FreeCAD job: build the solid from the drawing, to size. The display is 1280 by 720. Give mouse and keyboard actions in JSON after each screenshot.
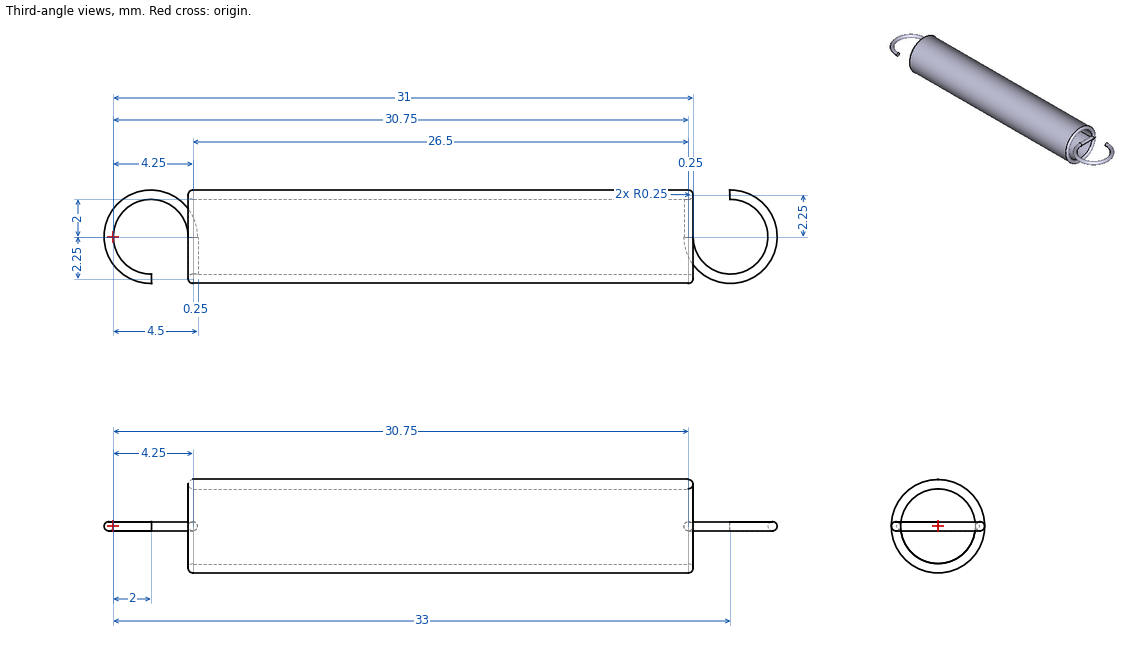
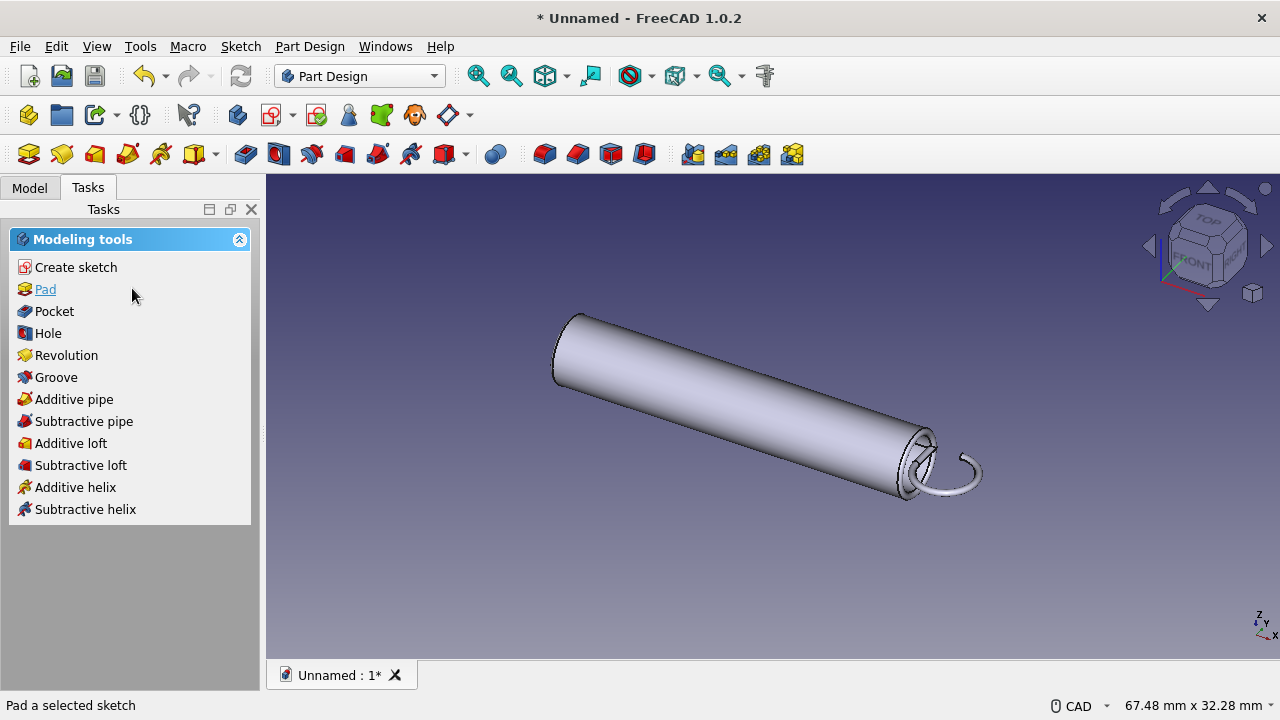
{"action": "left_click", "coordinate": [62, 154]}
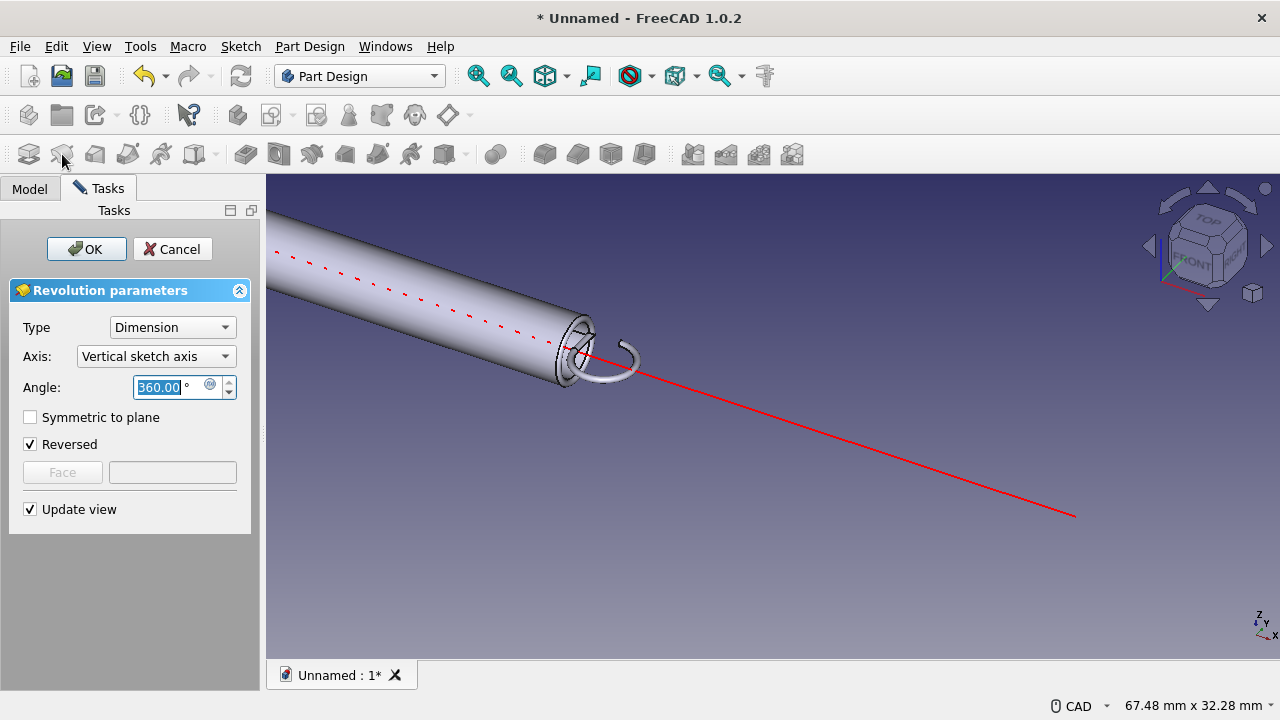
{"action": "left_click", "coordinate": [157, 356]}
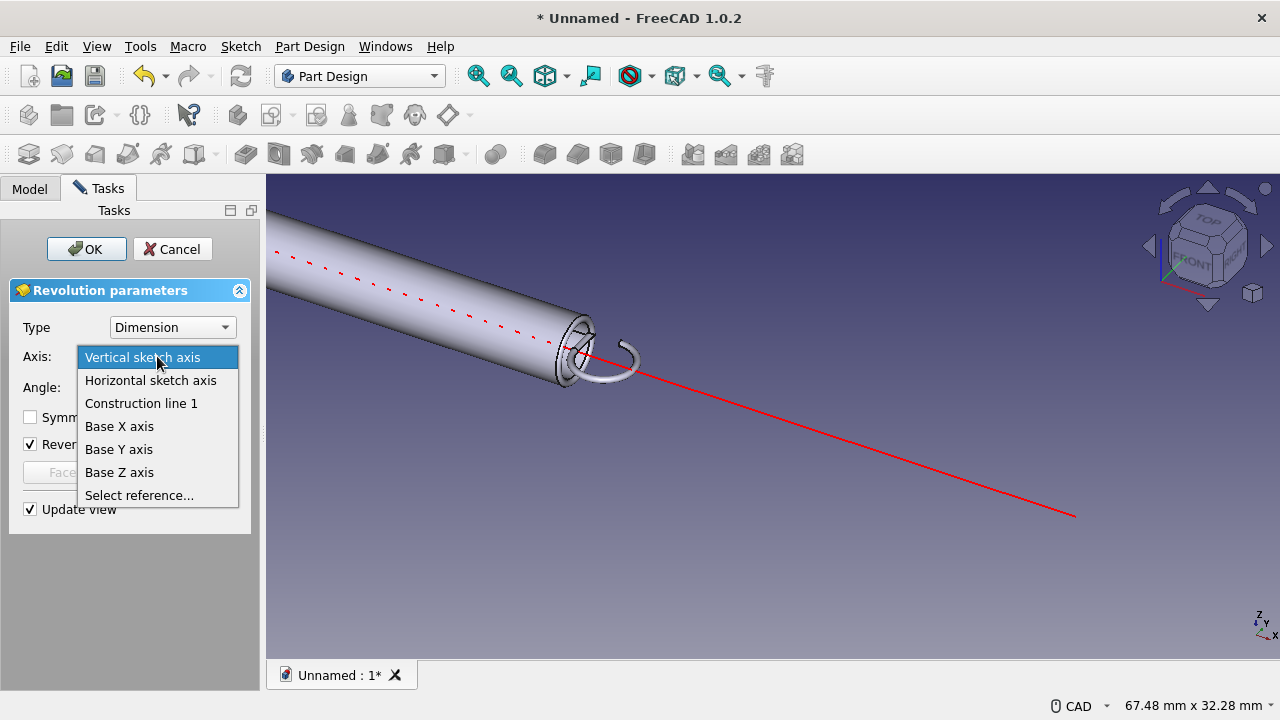
{"action": "left_click", "coordinate": [156, 404]}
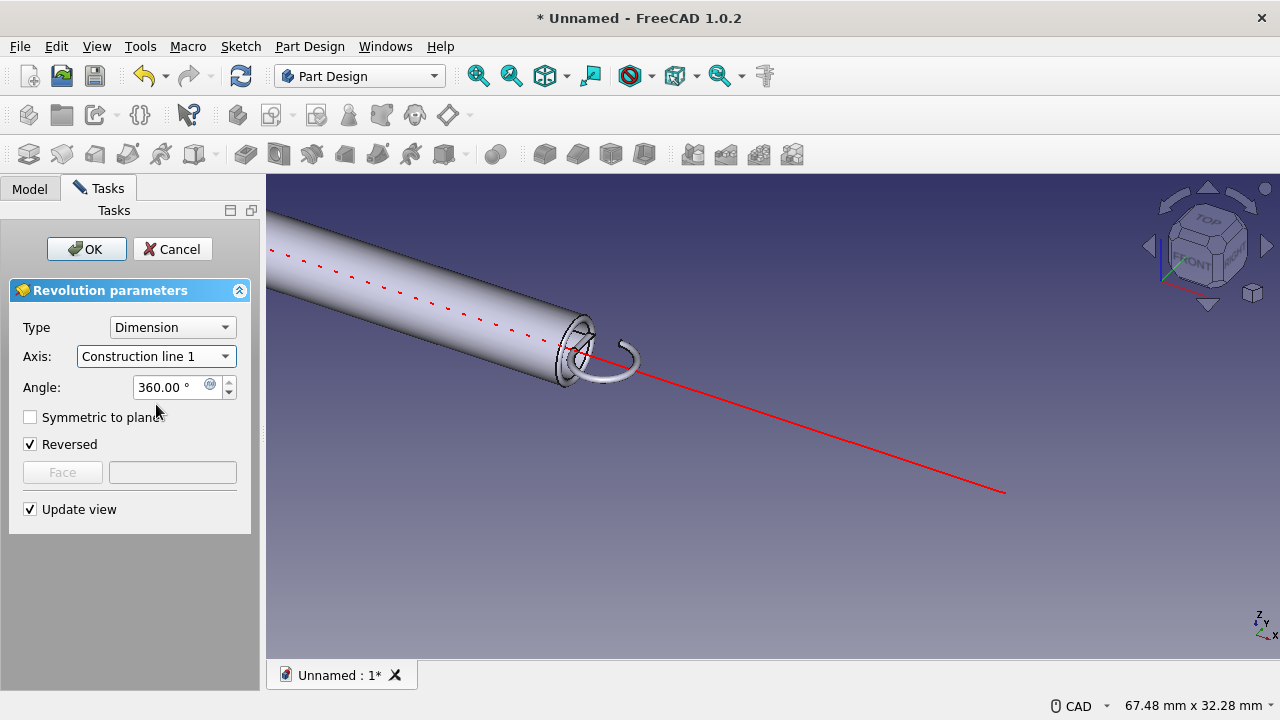
{"action": "triple_click", "coordinate": [178, 388]}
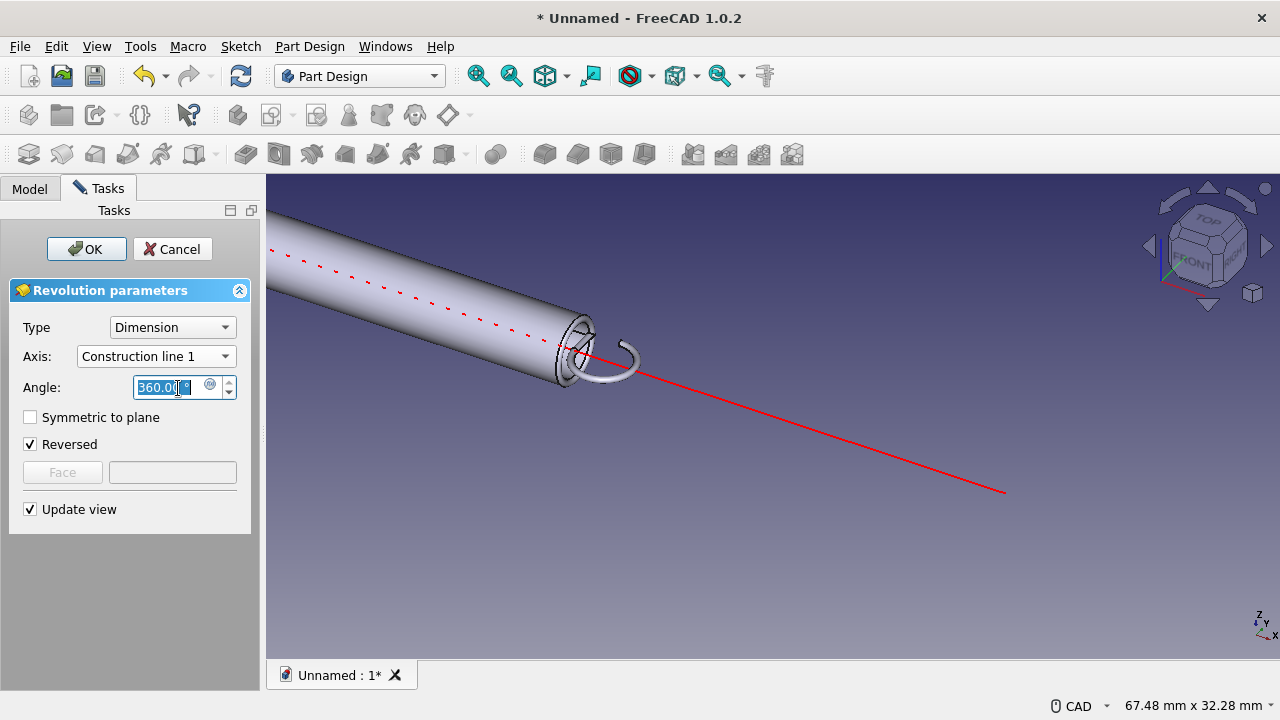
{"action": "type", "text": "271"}
{"action": "key", "text": "Tab"}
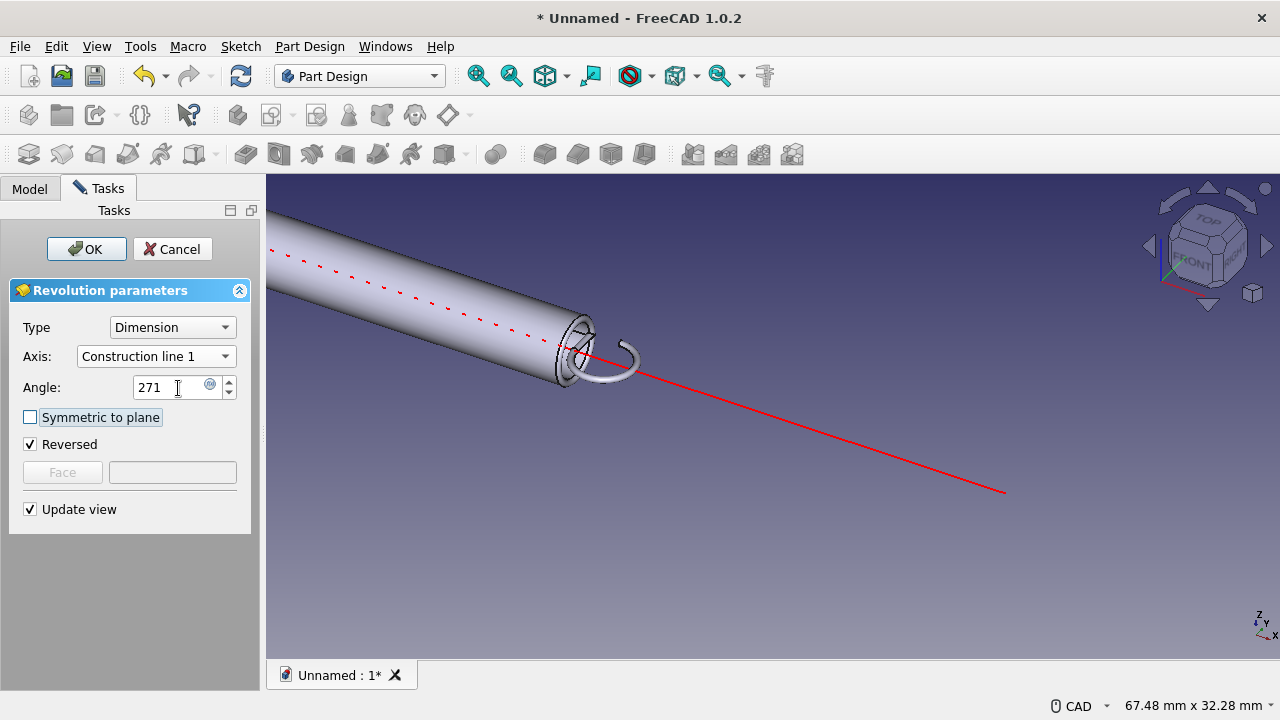
{"action": "left_click", "coordinate": [31, 444]}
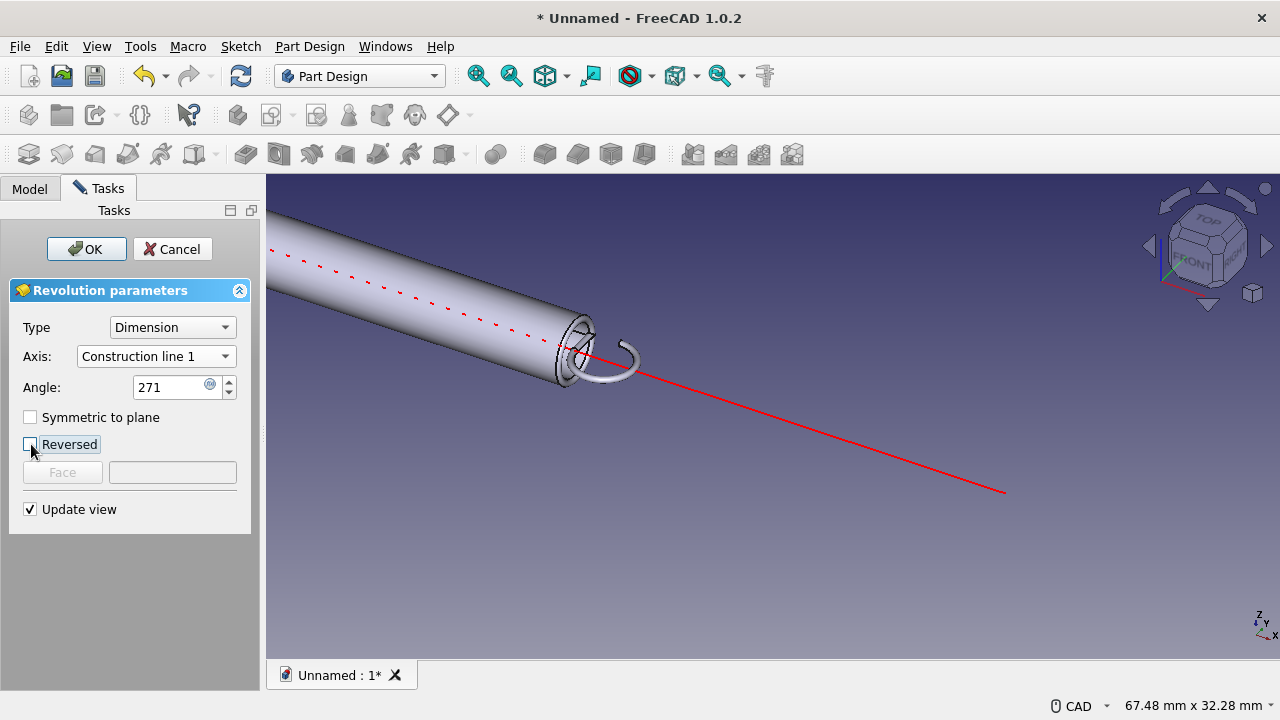
{"action": "left_click", "coordinate": [87, 249]}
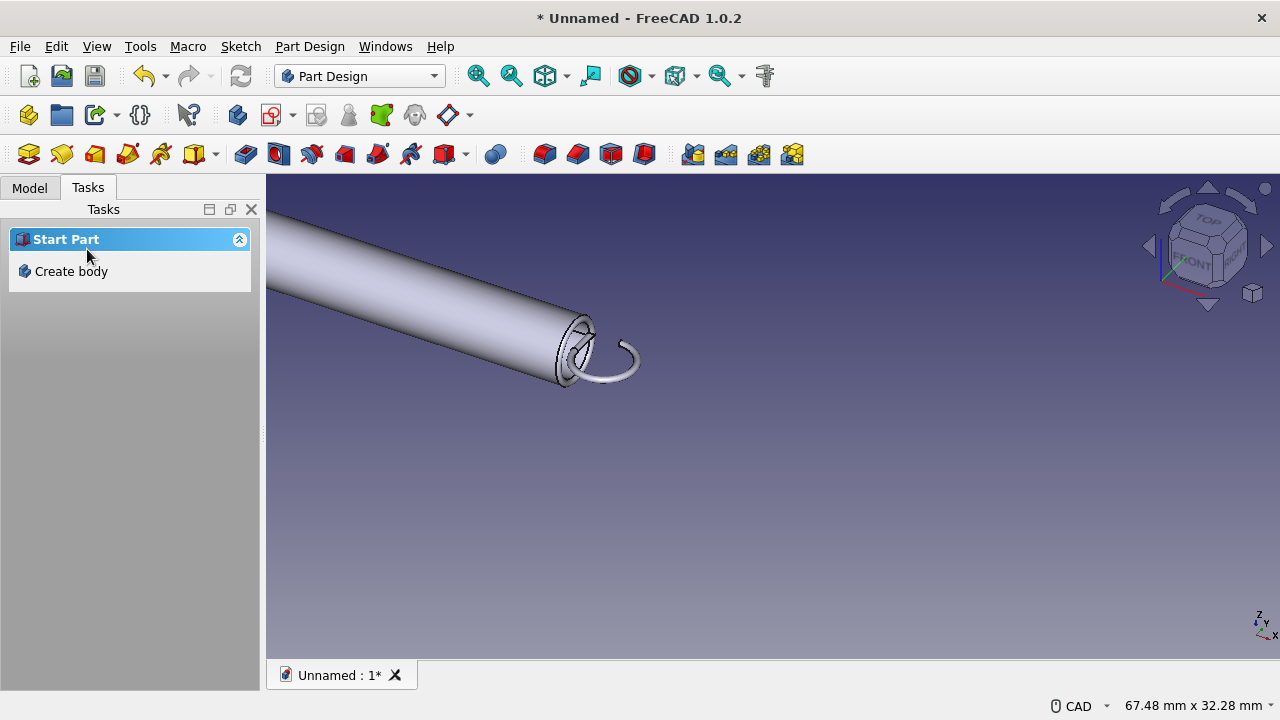
{"action": "key", "text": "0"}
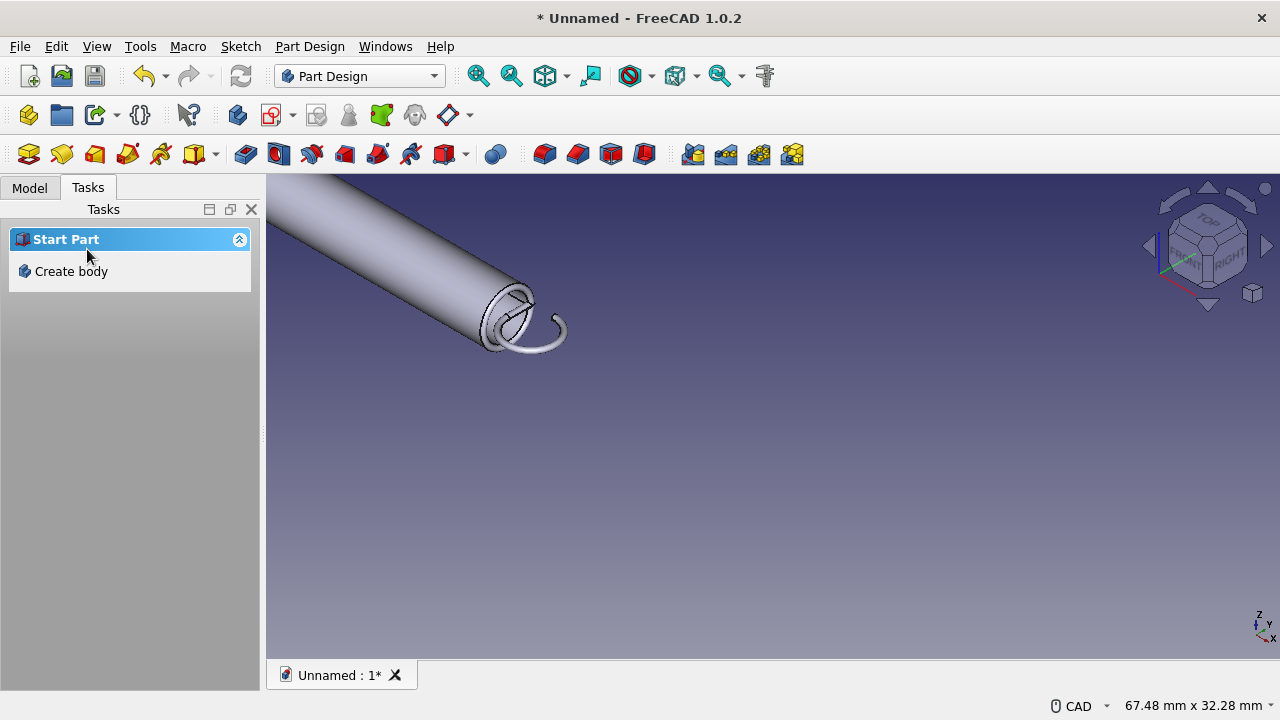
{"action": "key", "text": "v f"}